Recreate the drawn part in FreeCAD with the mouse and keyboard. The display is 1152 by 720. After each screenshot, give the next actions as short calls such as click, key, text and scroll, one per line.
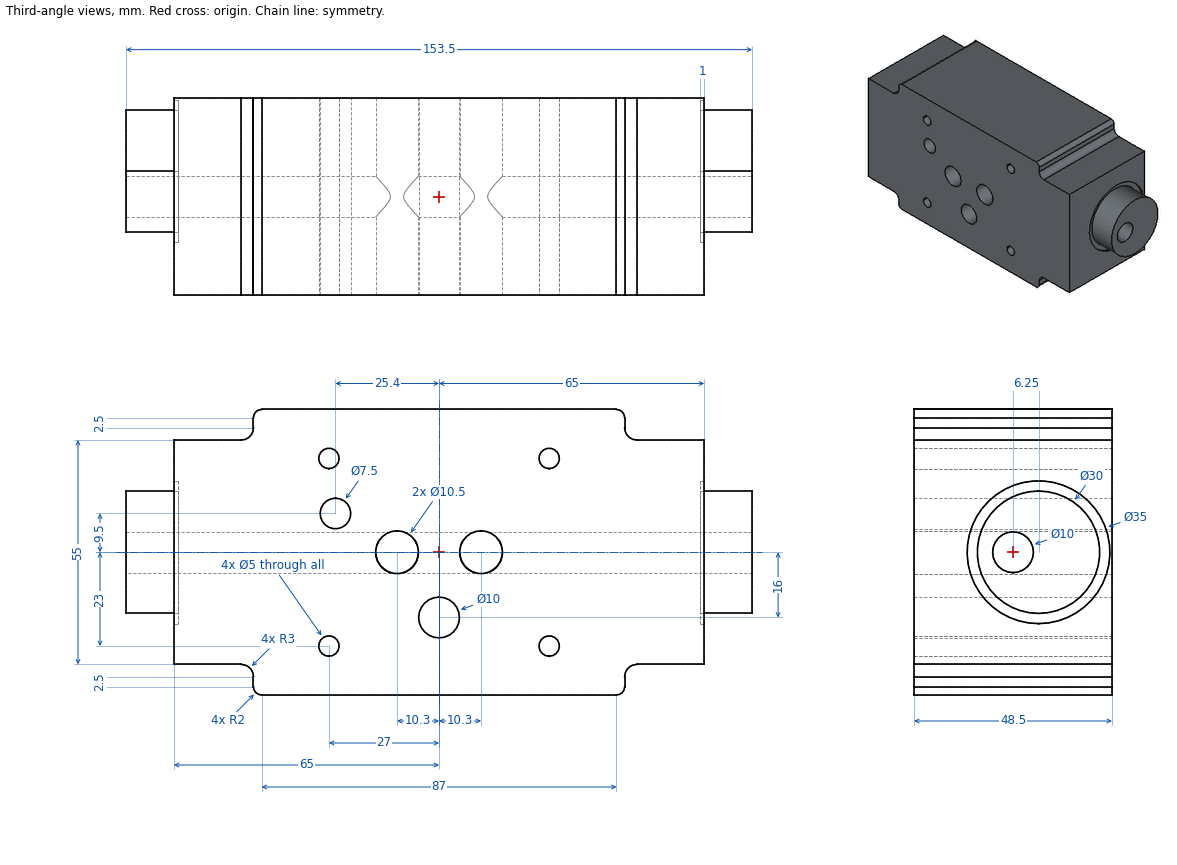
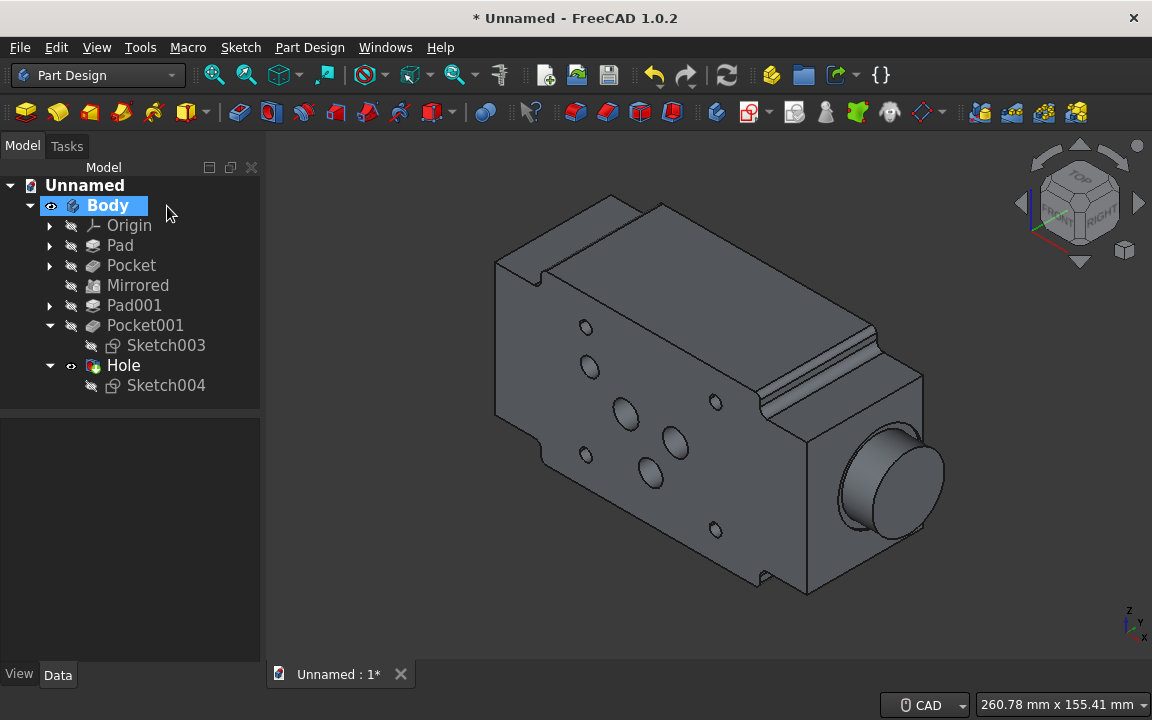
click(908, 492)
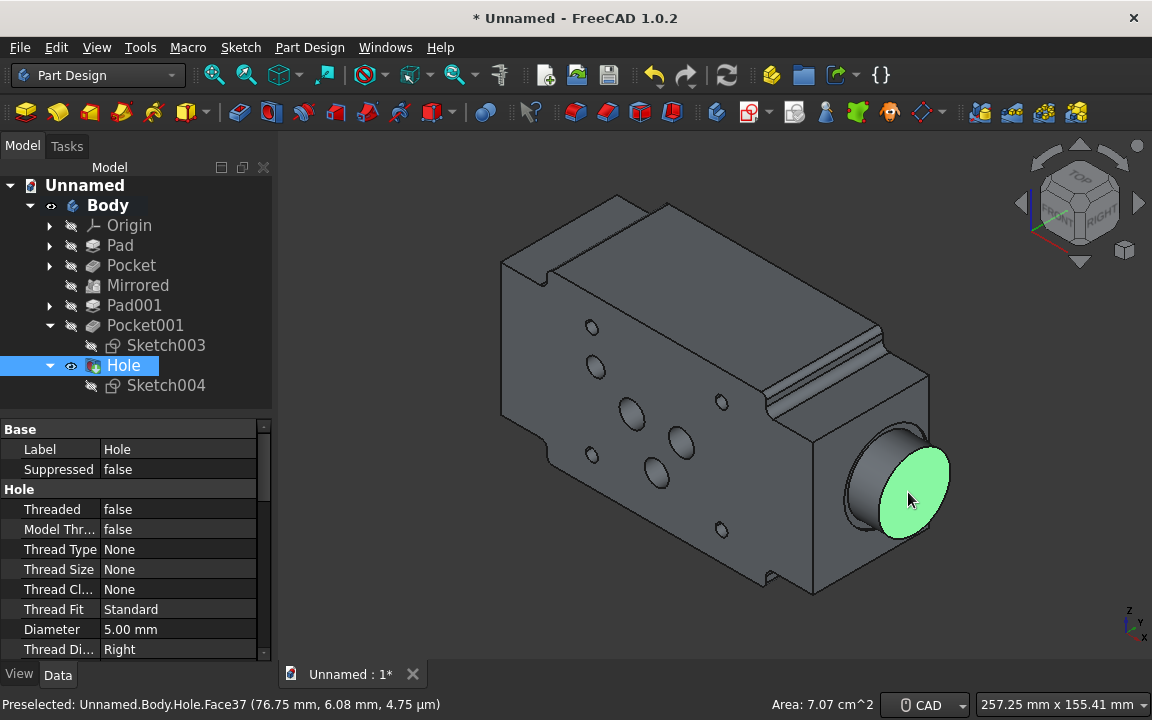
click(750, 112)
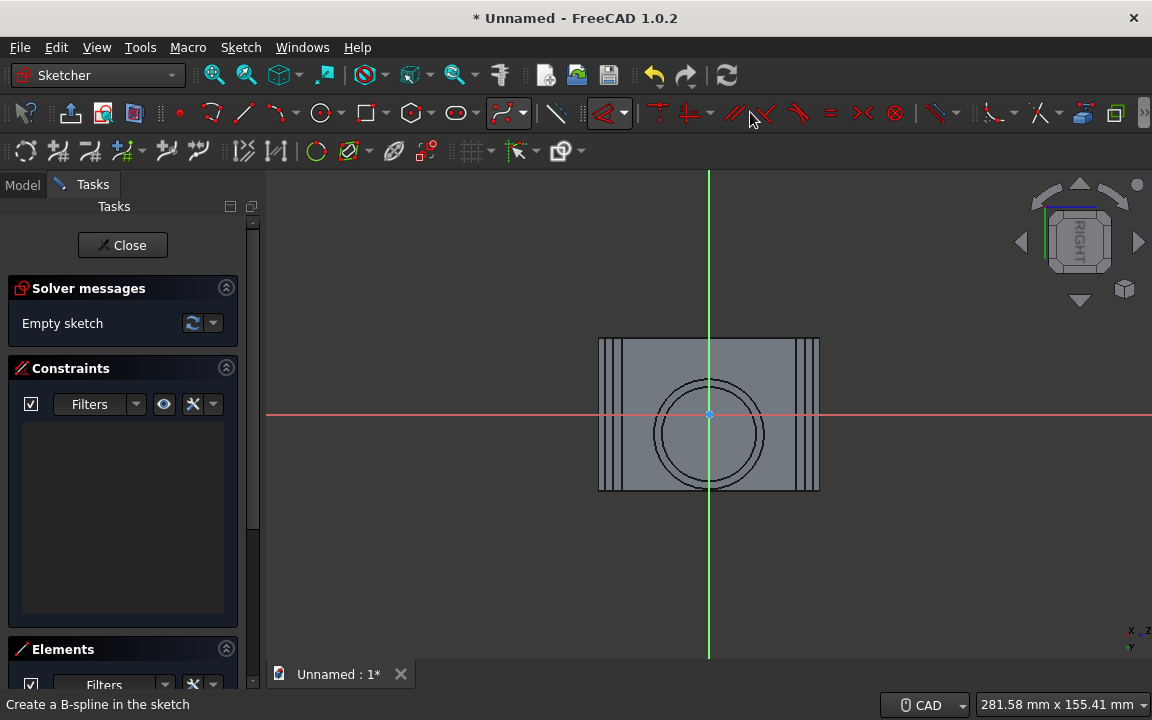
scroll(718, 415, up, 11)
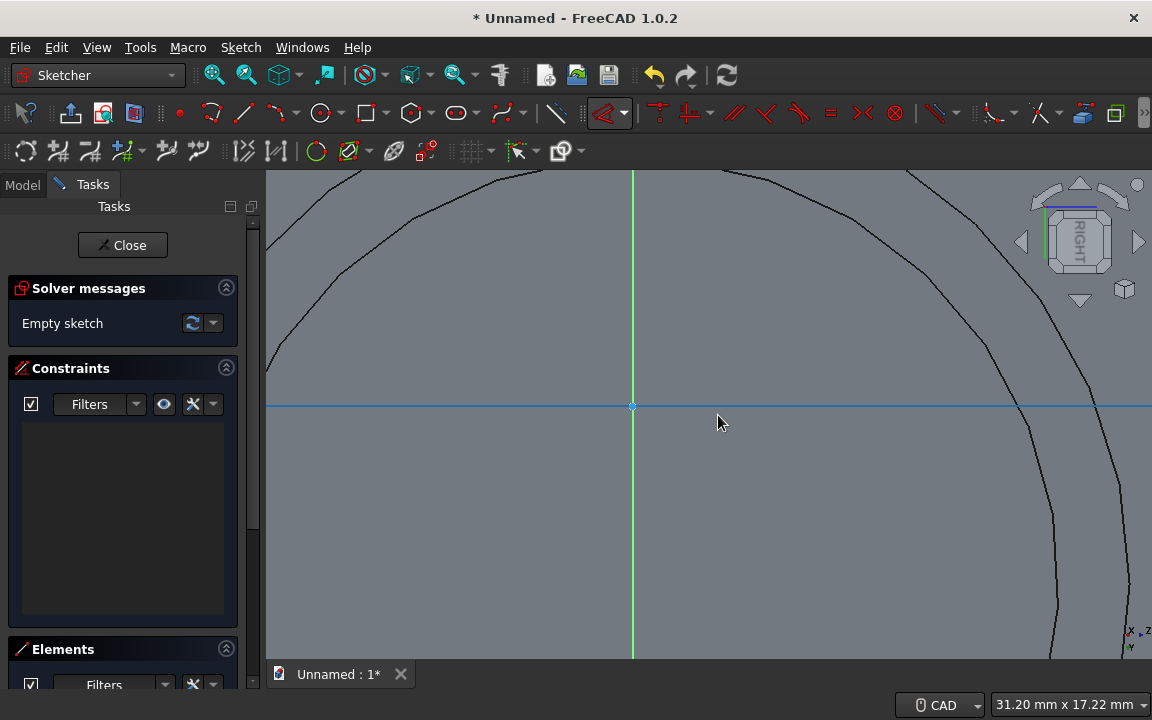
click(322, 114)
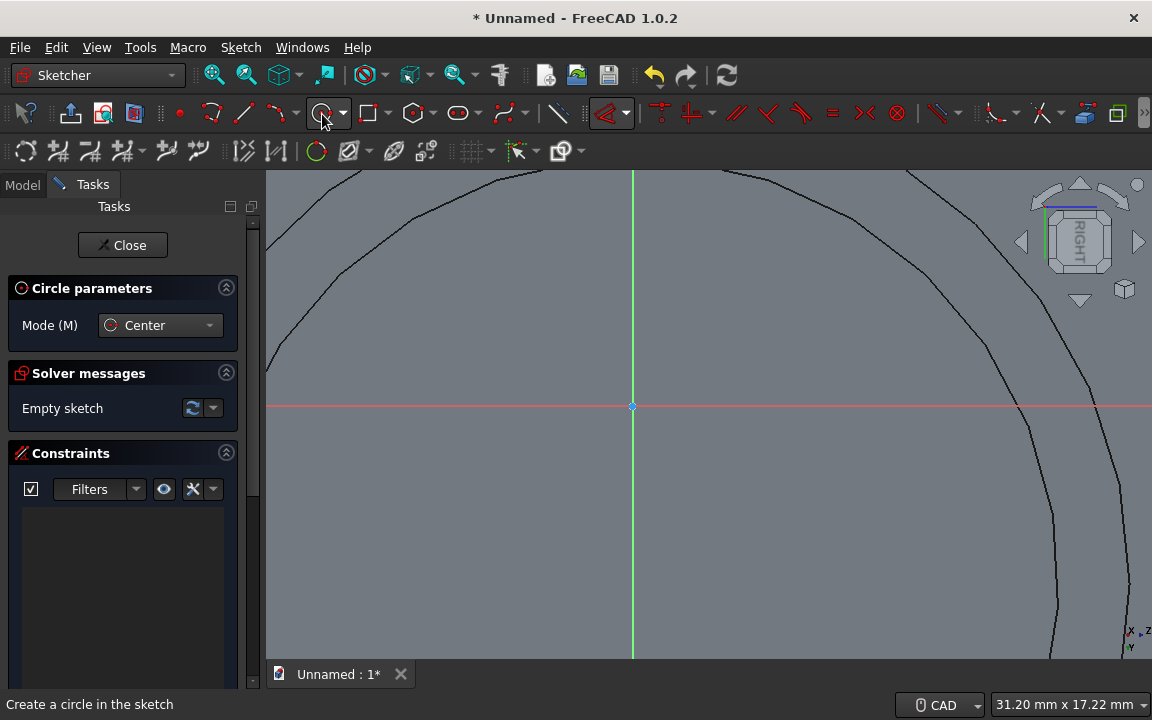
click(633, 406)
move(733, 306)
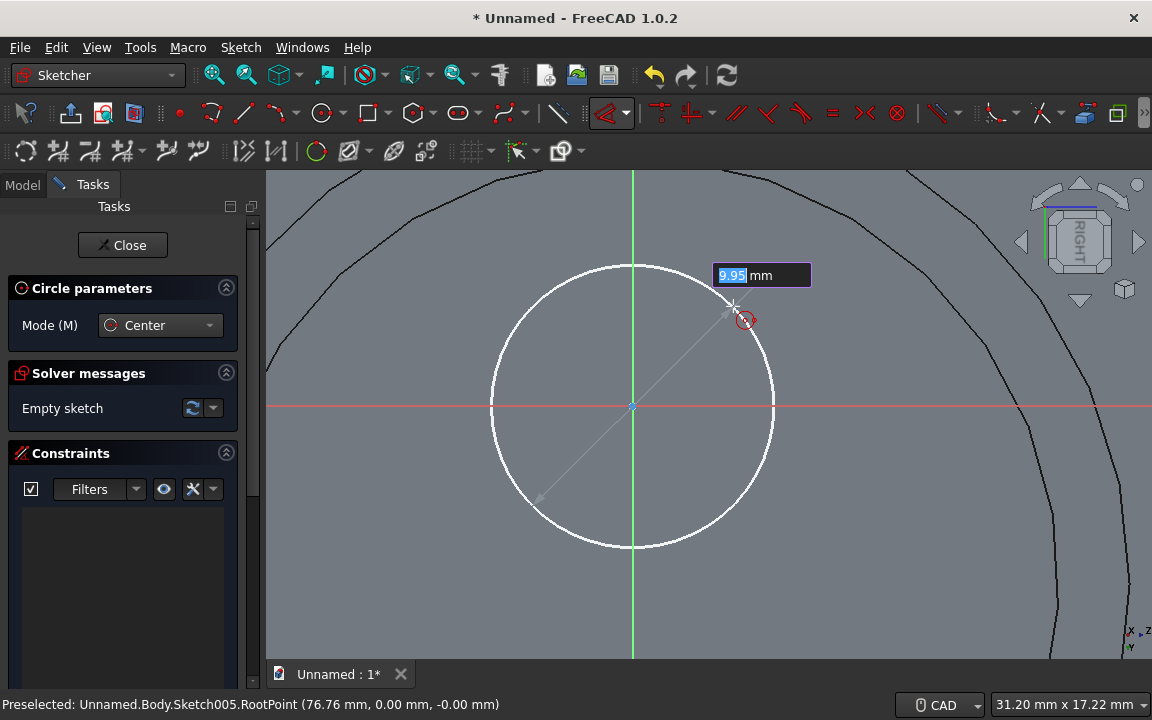
text(10)
key(Return)
key(Escape)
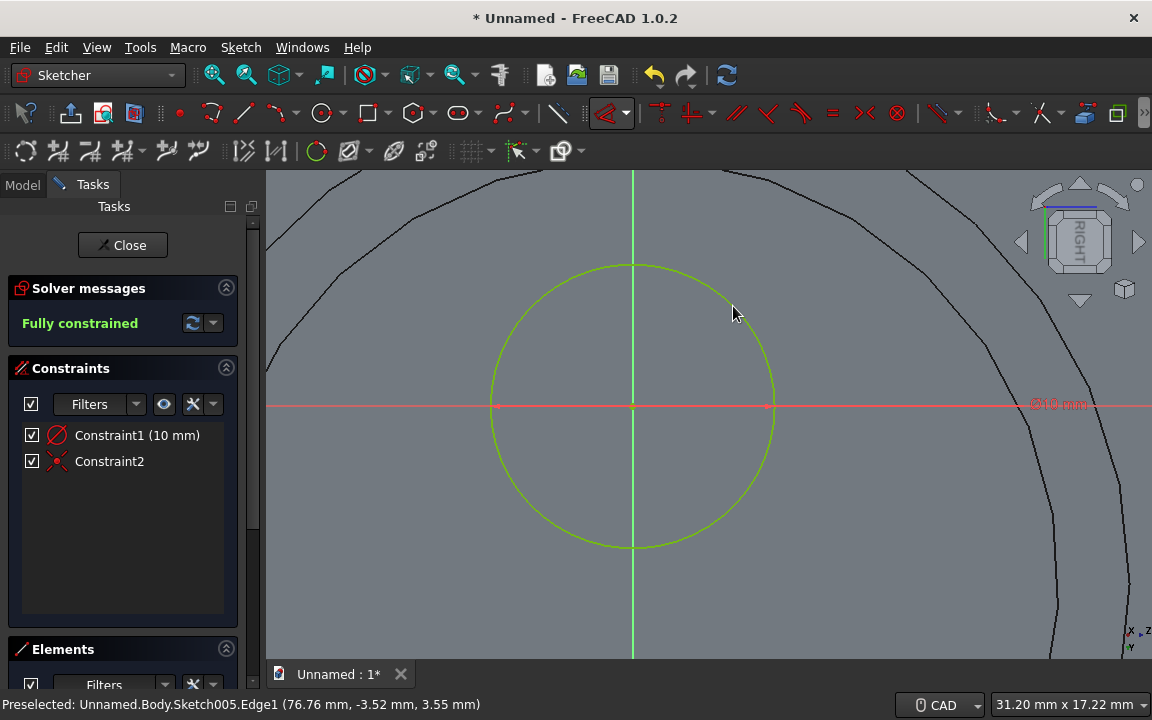
click(123, 245)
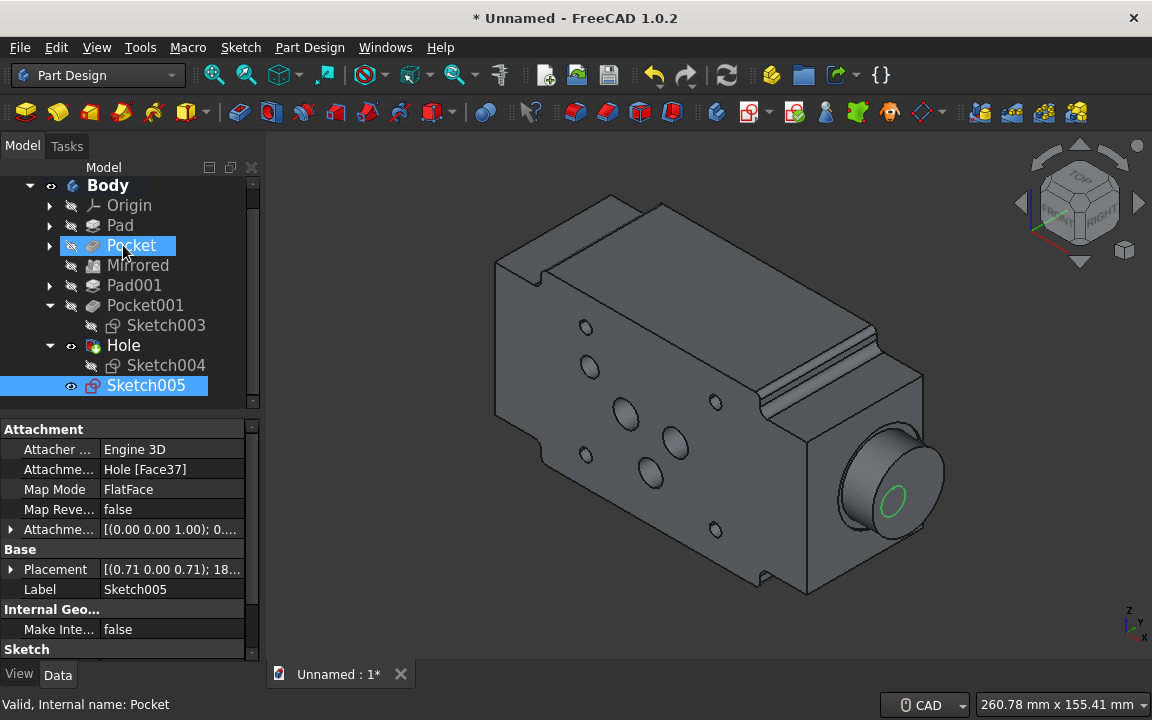
click(240, 112)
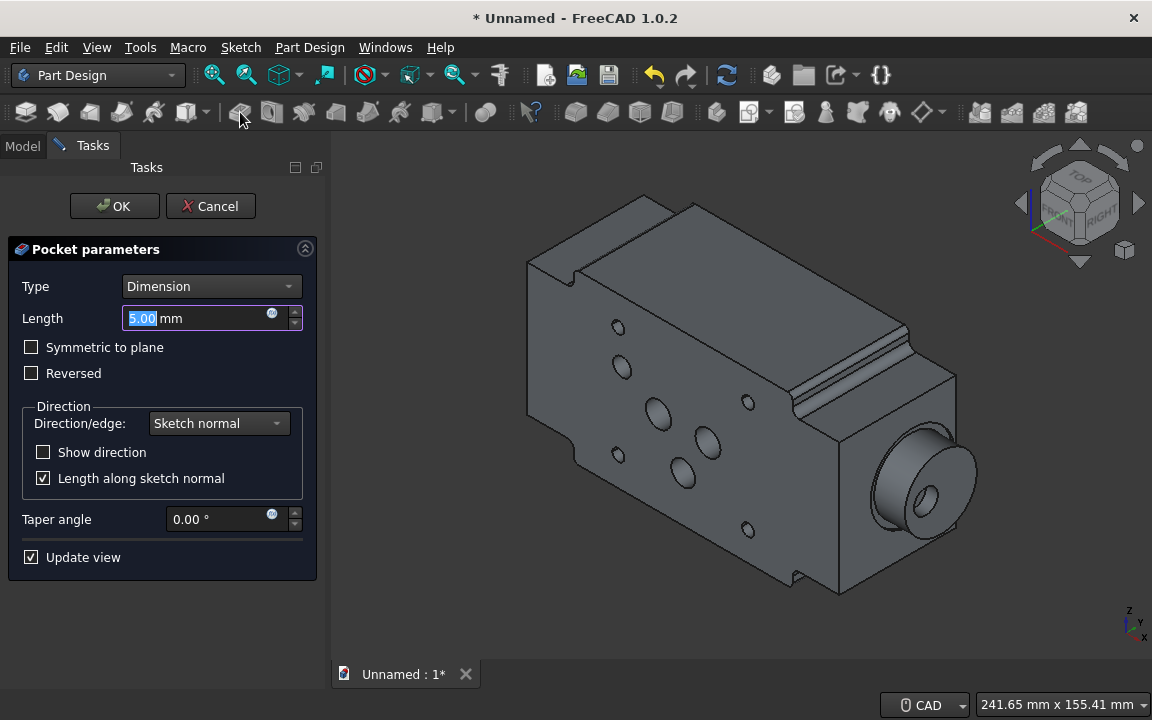
click(212, 286)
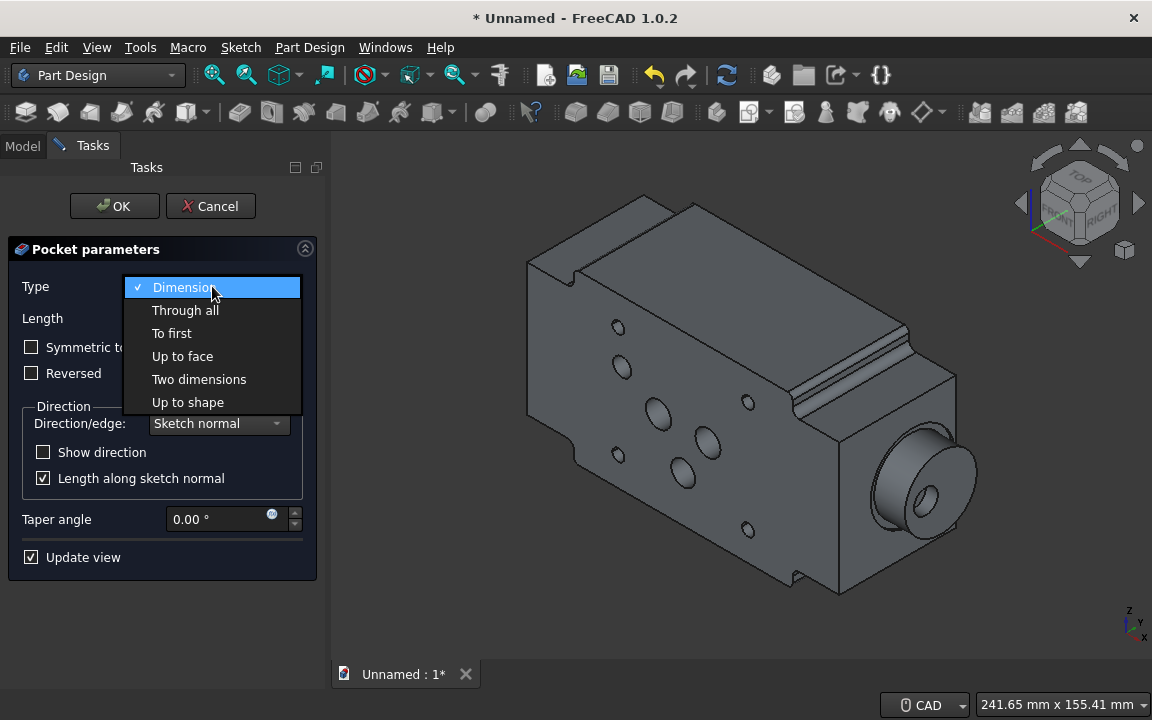
click(212, 310)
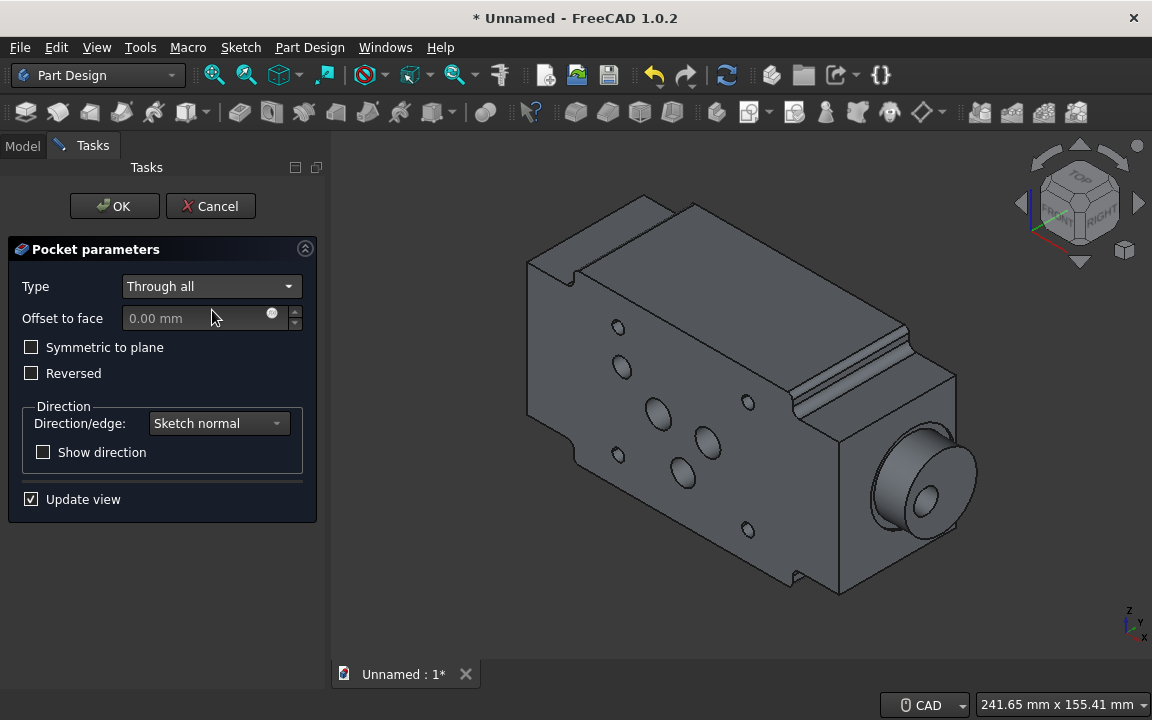
click(115, 206)